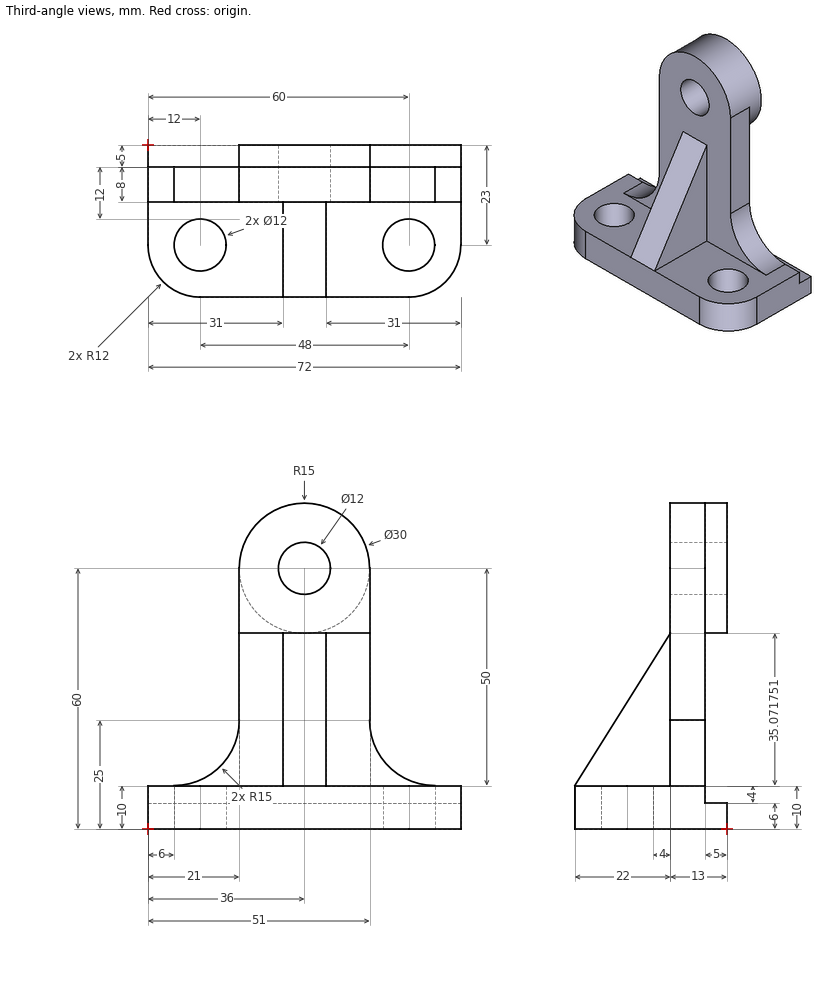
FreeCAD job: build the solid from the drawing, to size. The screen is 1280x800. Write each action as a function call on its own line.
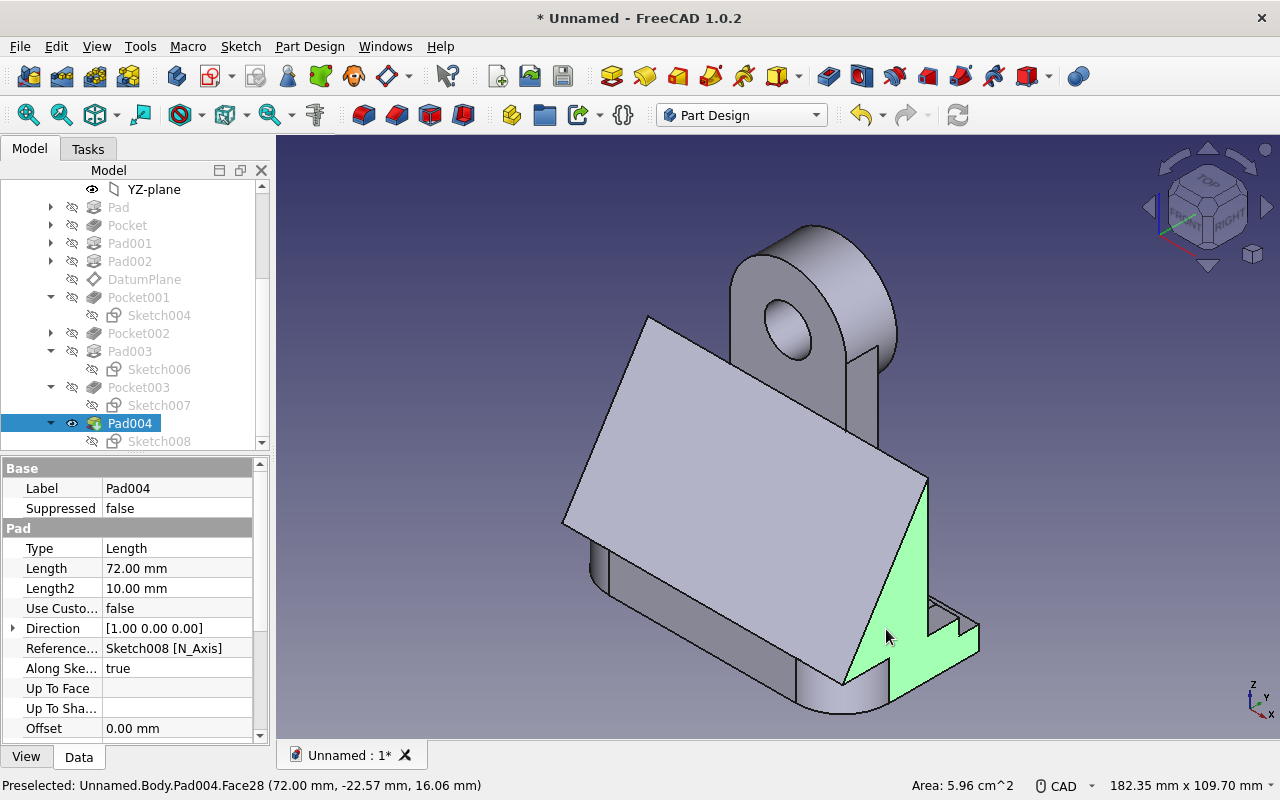
click(210, 76)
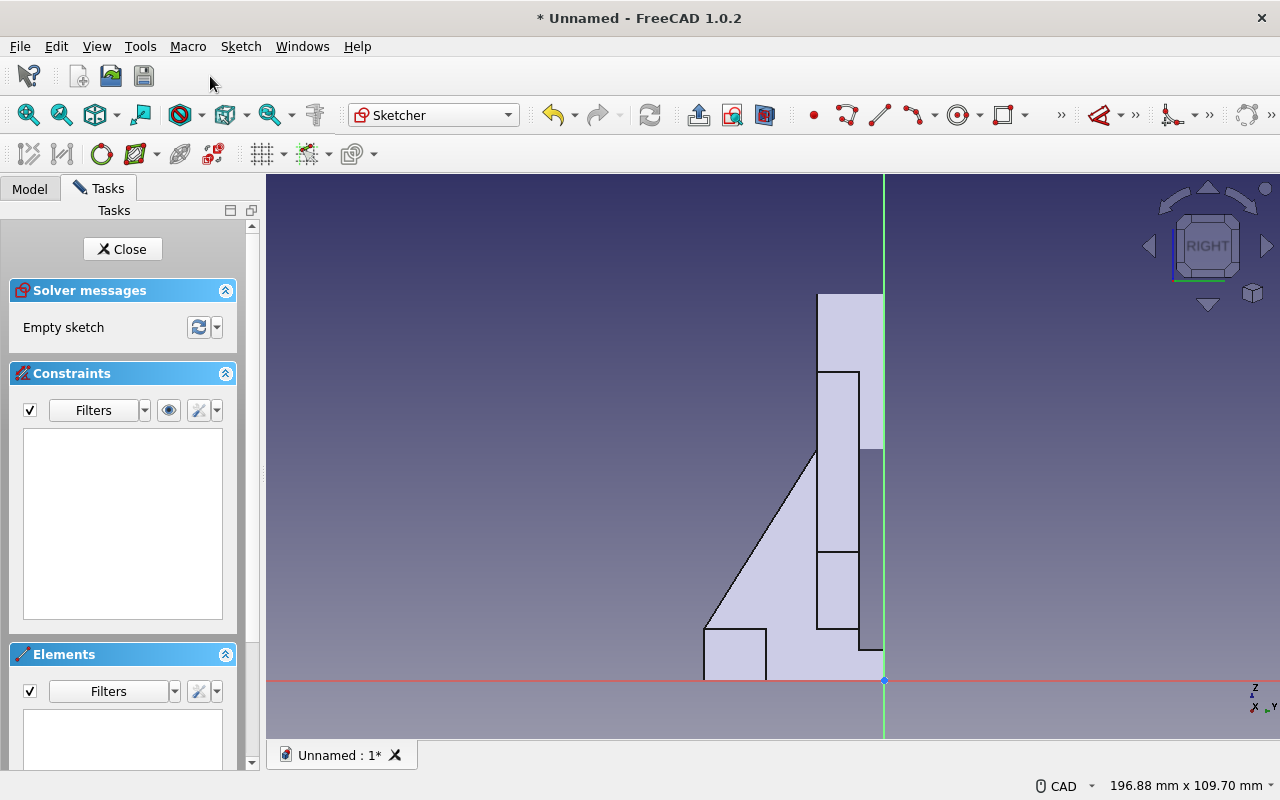
scroll(977, 711, up, 2)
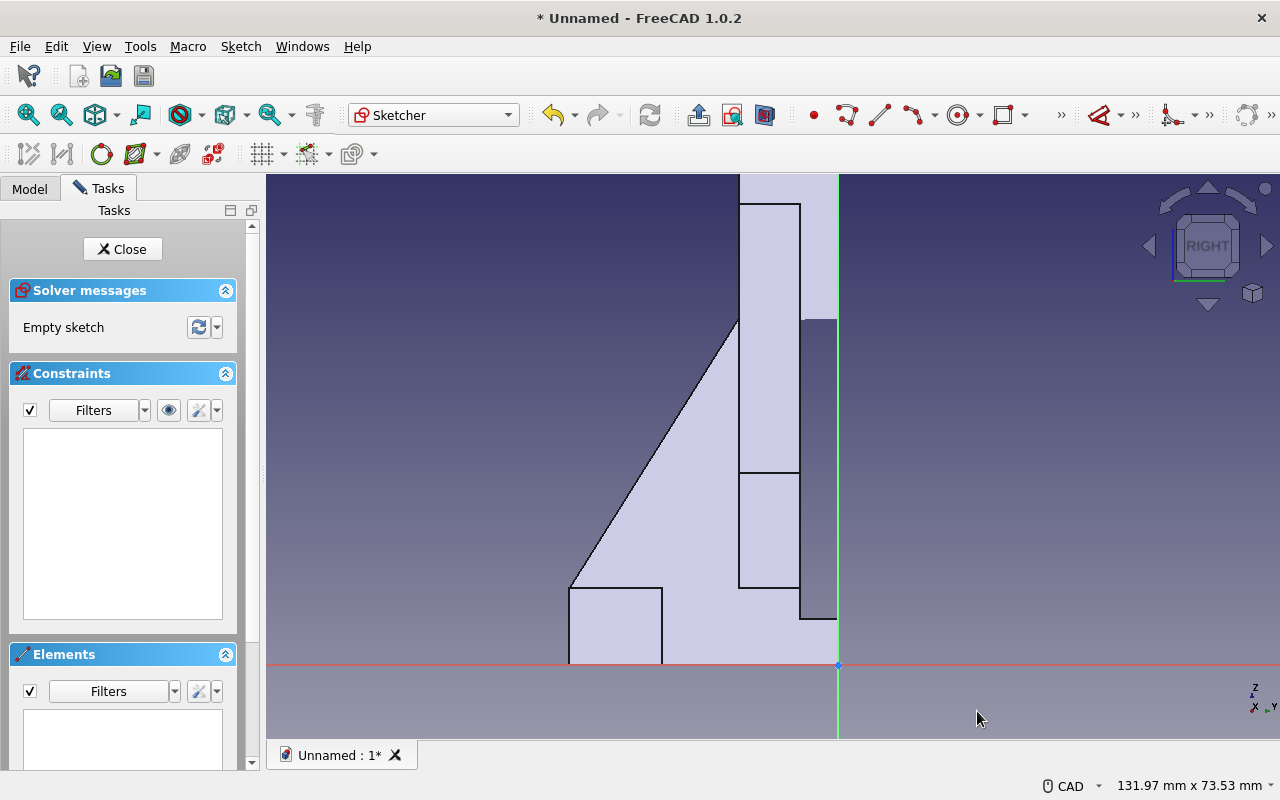
click(847, 116)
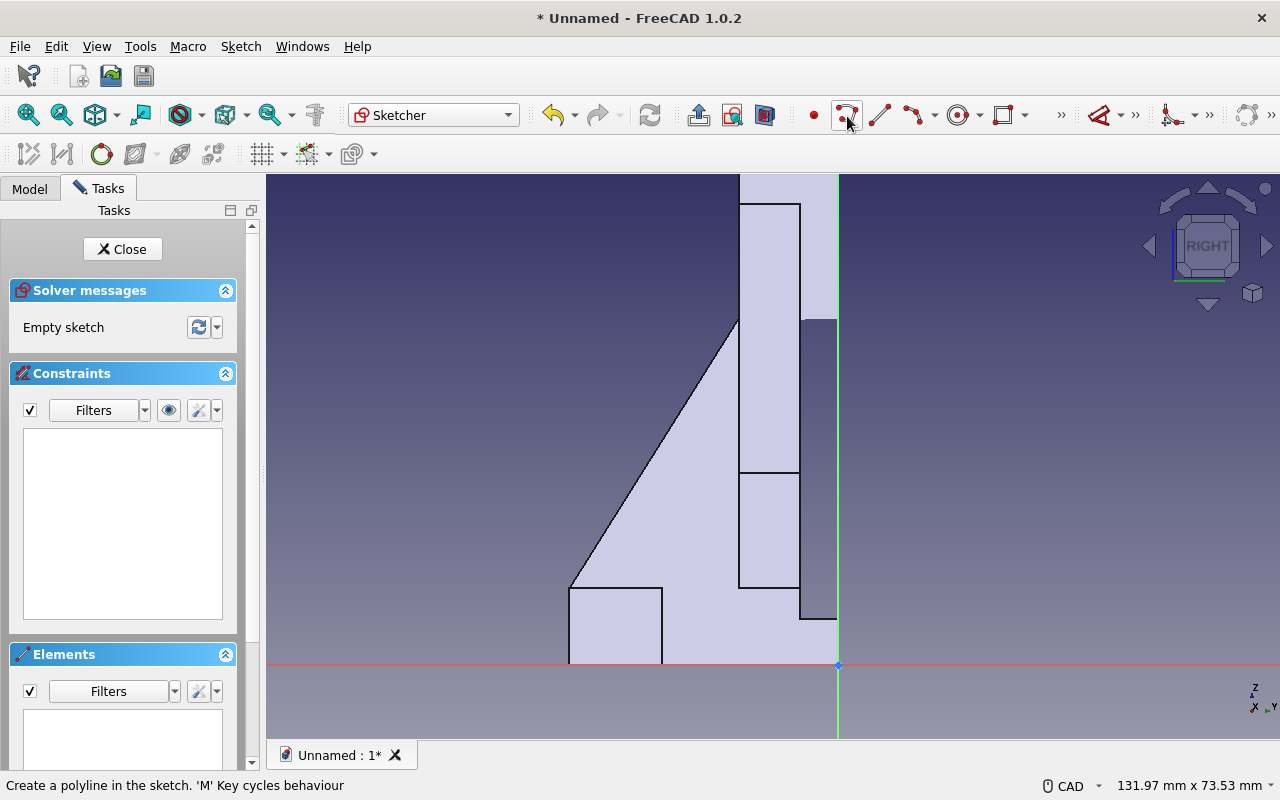
click(739, 588)
click(739, 319)
click(569, 588)
click(739, 589)
key(Escape)
key(Escape)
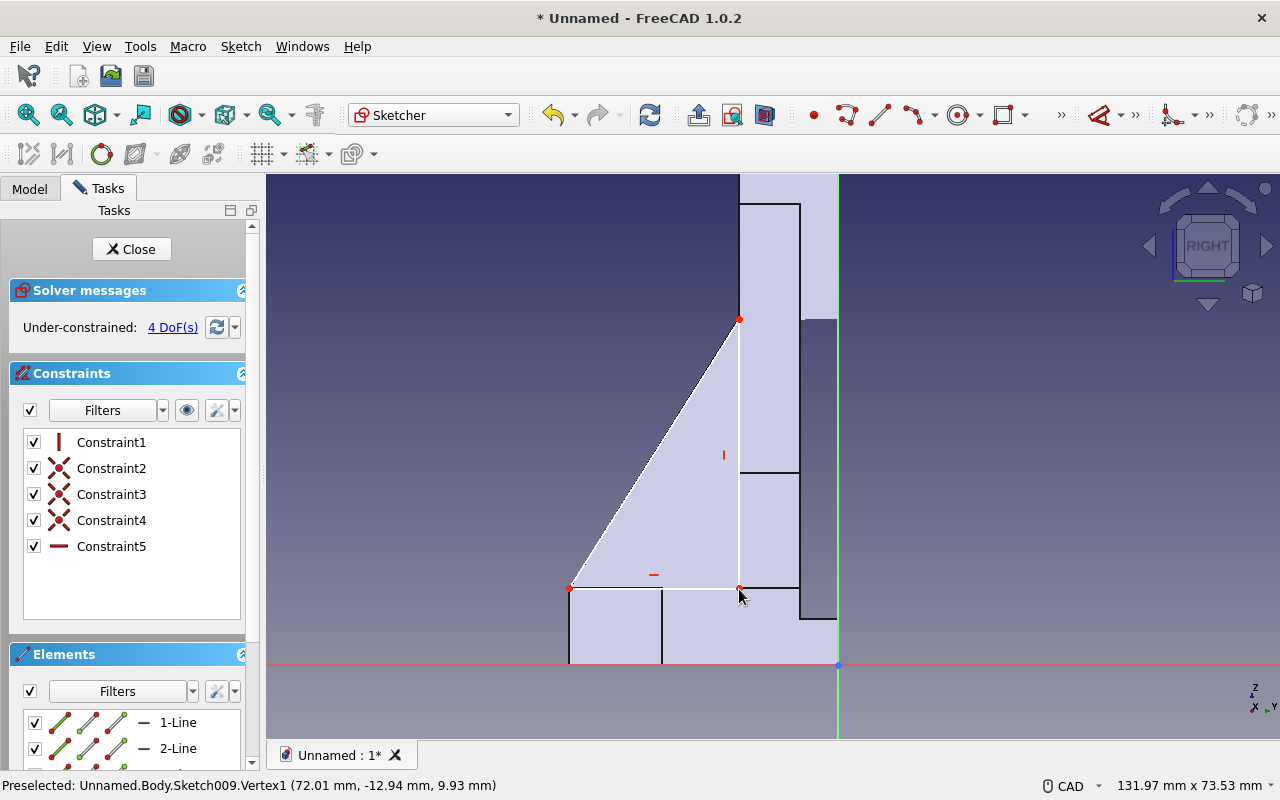
click(1098, 116)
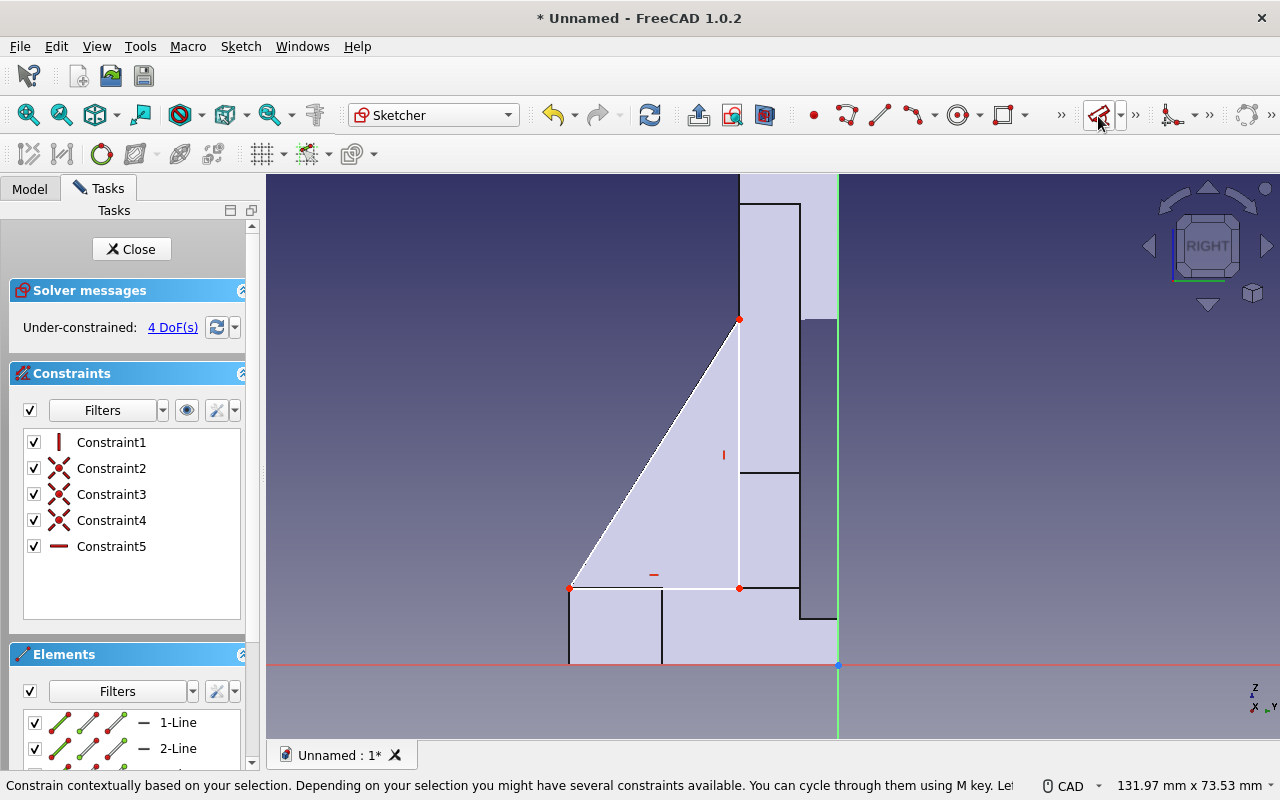
click(620, 589)
click(654, 623)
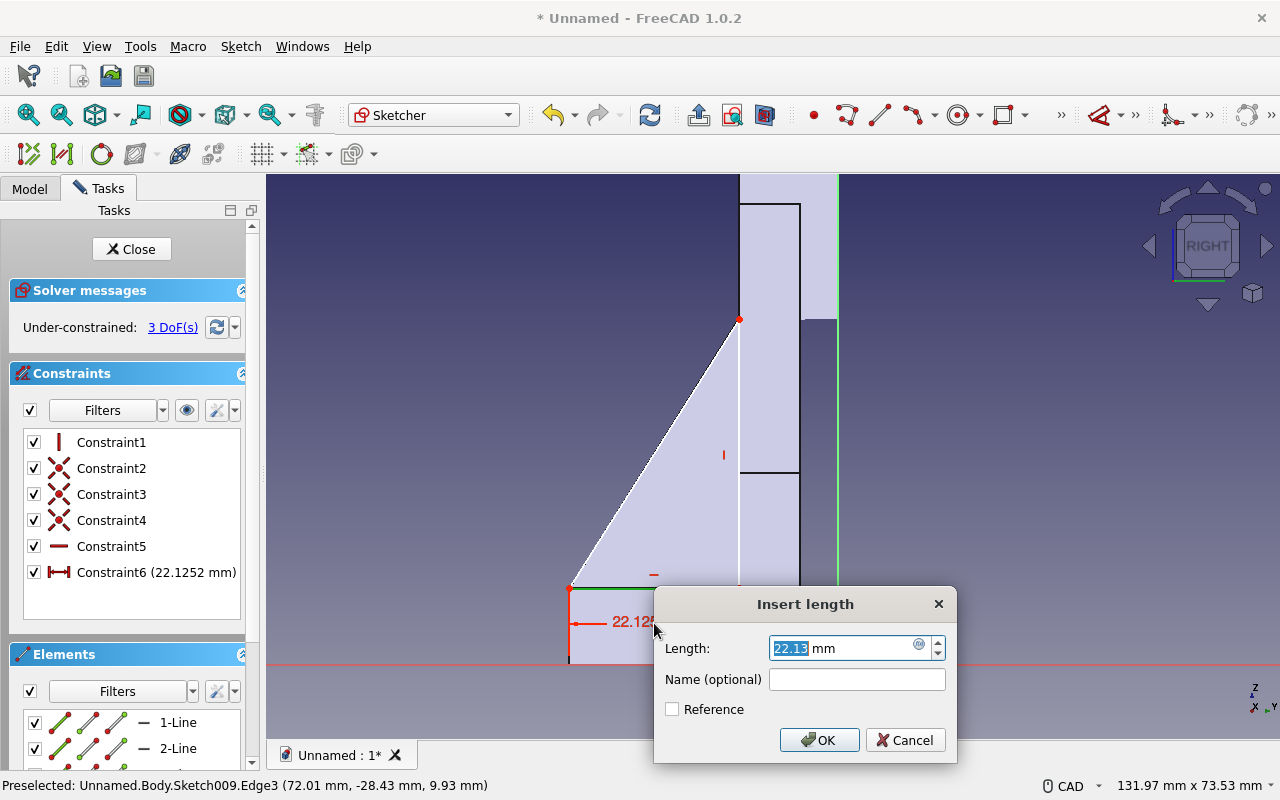
text(22)
key(Return)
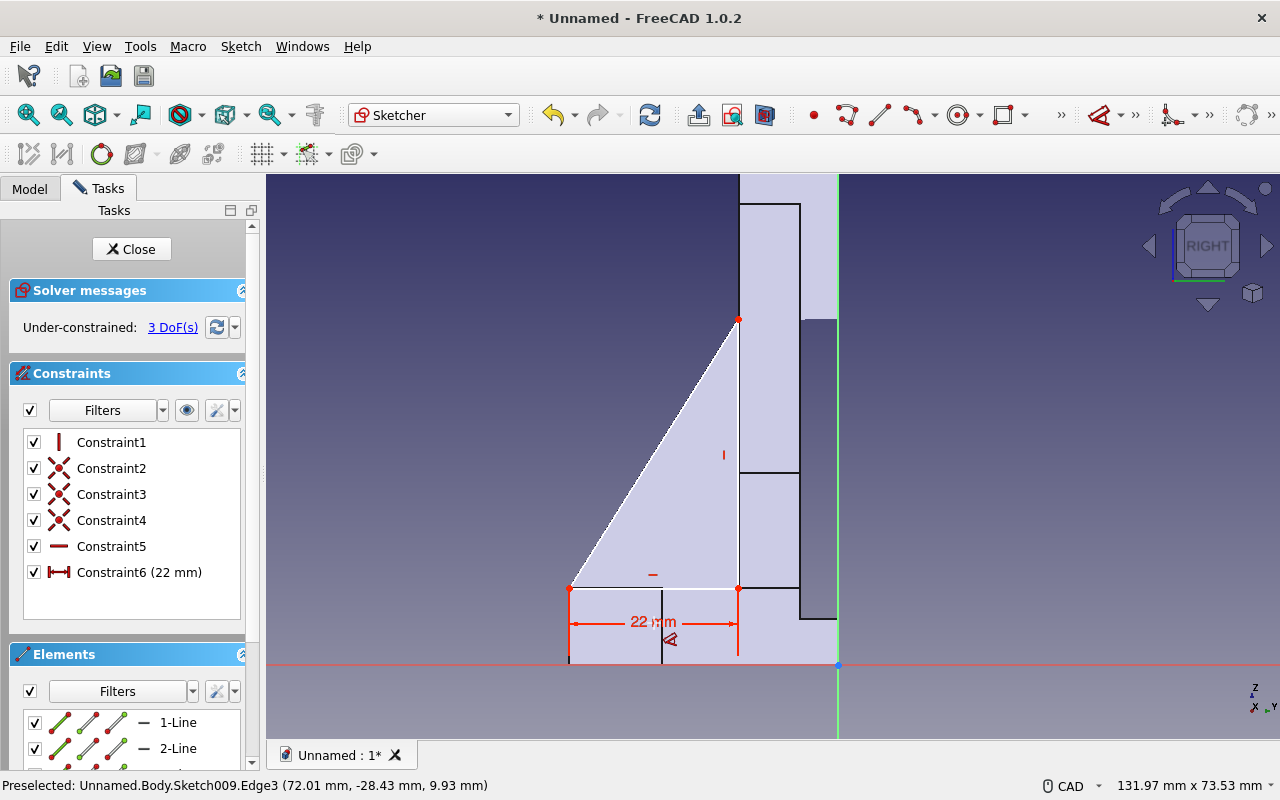
click(738, 589)
click(788, 699)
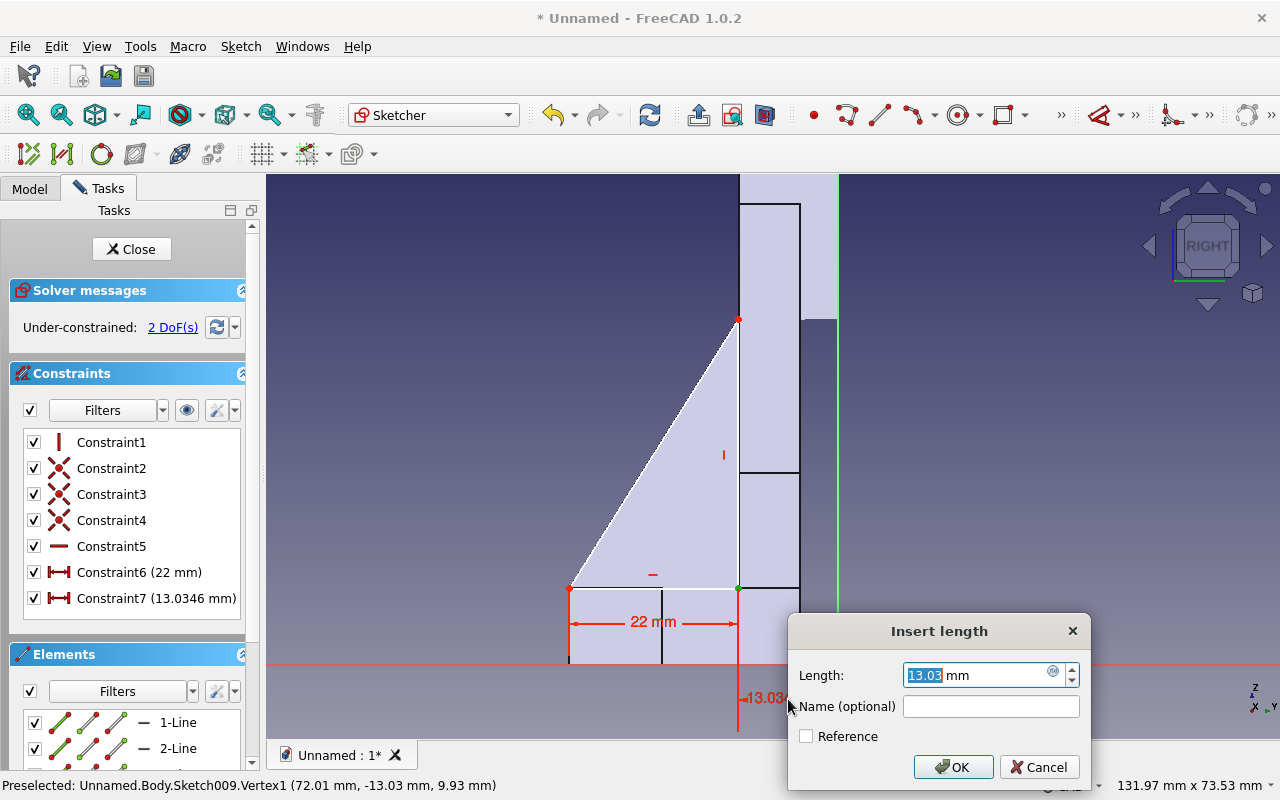
text(13)
key(Return)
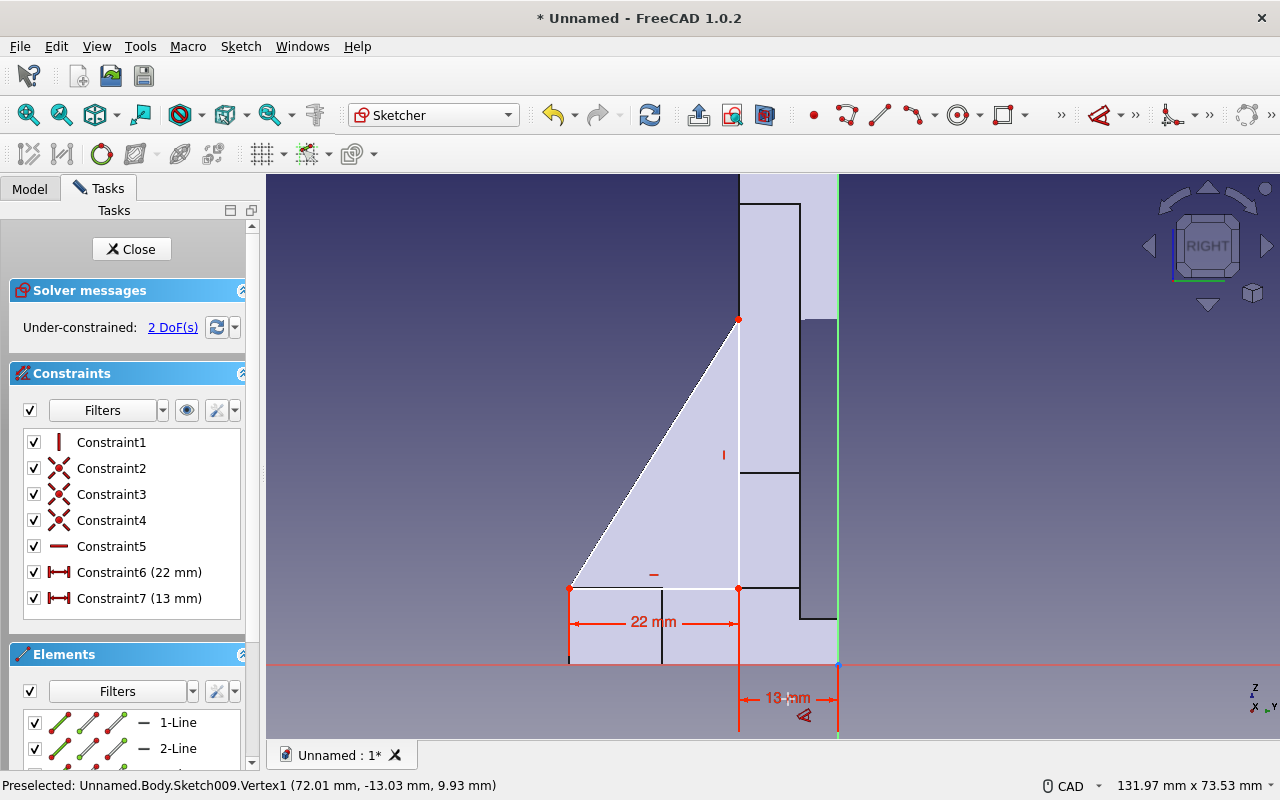
click(739, 589)
click(872, 627)